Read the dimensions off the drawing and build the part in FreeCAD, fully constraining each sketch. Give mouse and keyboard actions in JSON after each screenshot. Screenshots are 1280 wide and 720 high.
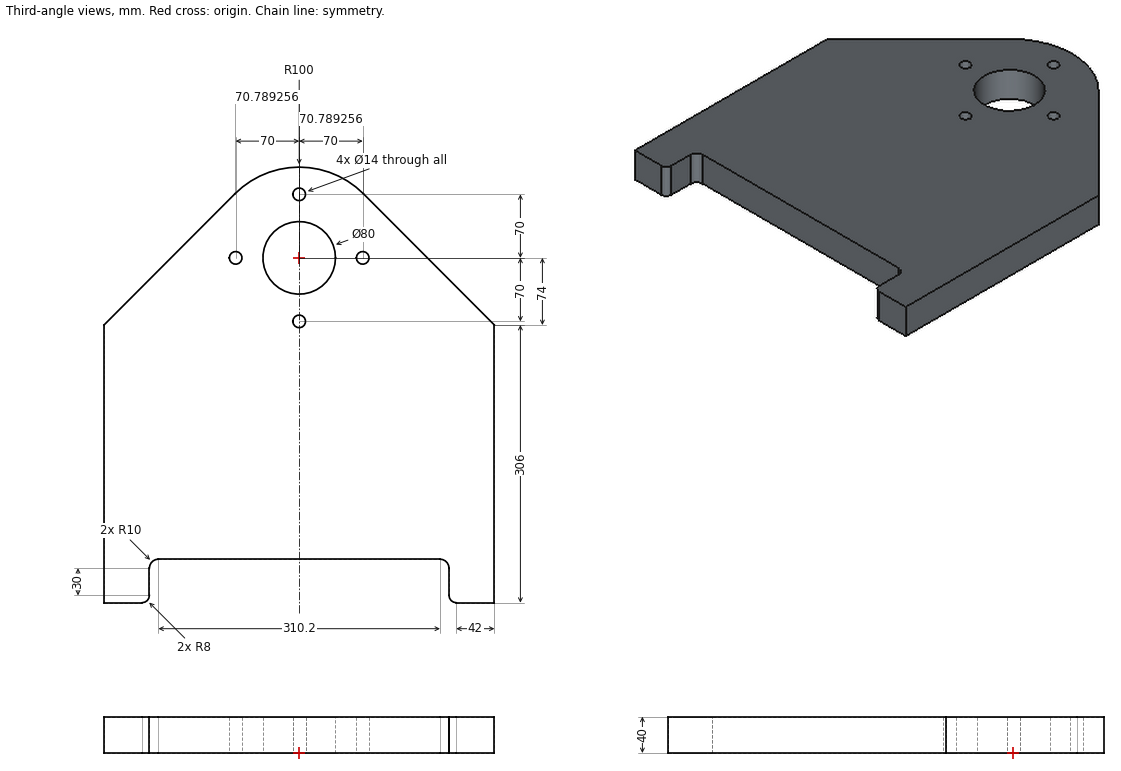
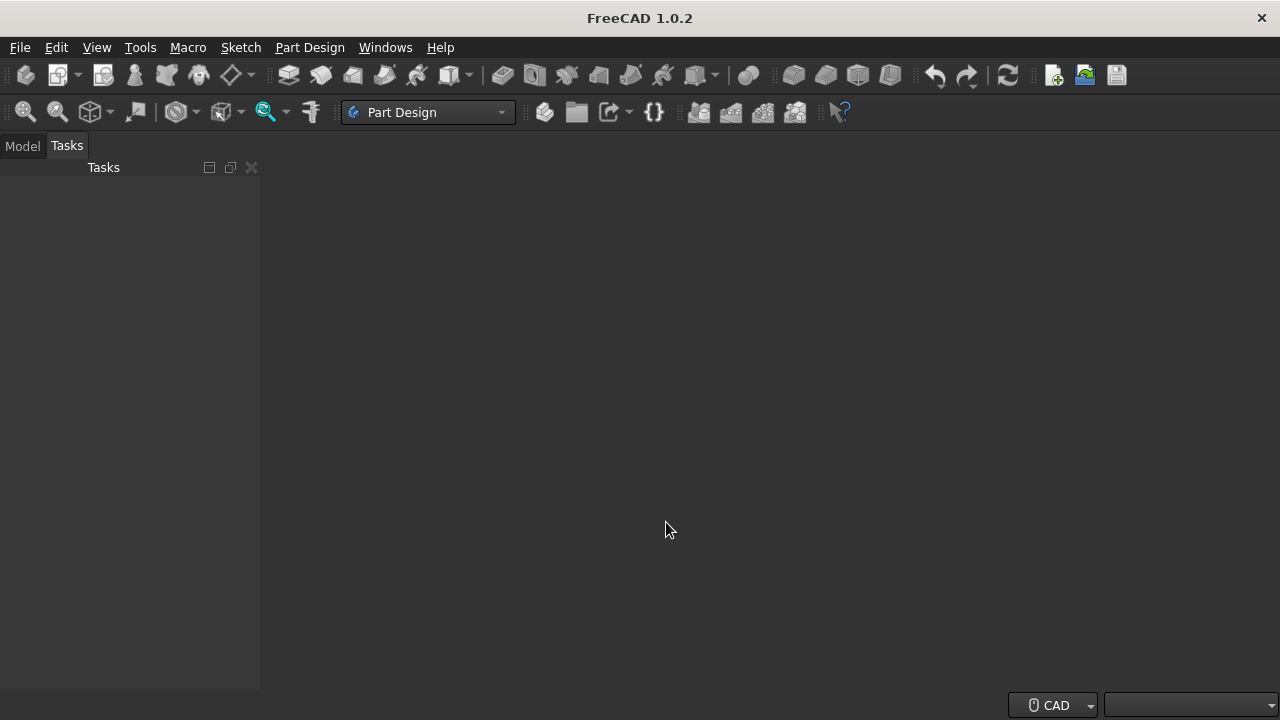
{"action": "key", "text": "ctrl+n"}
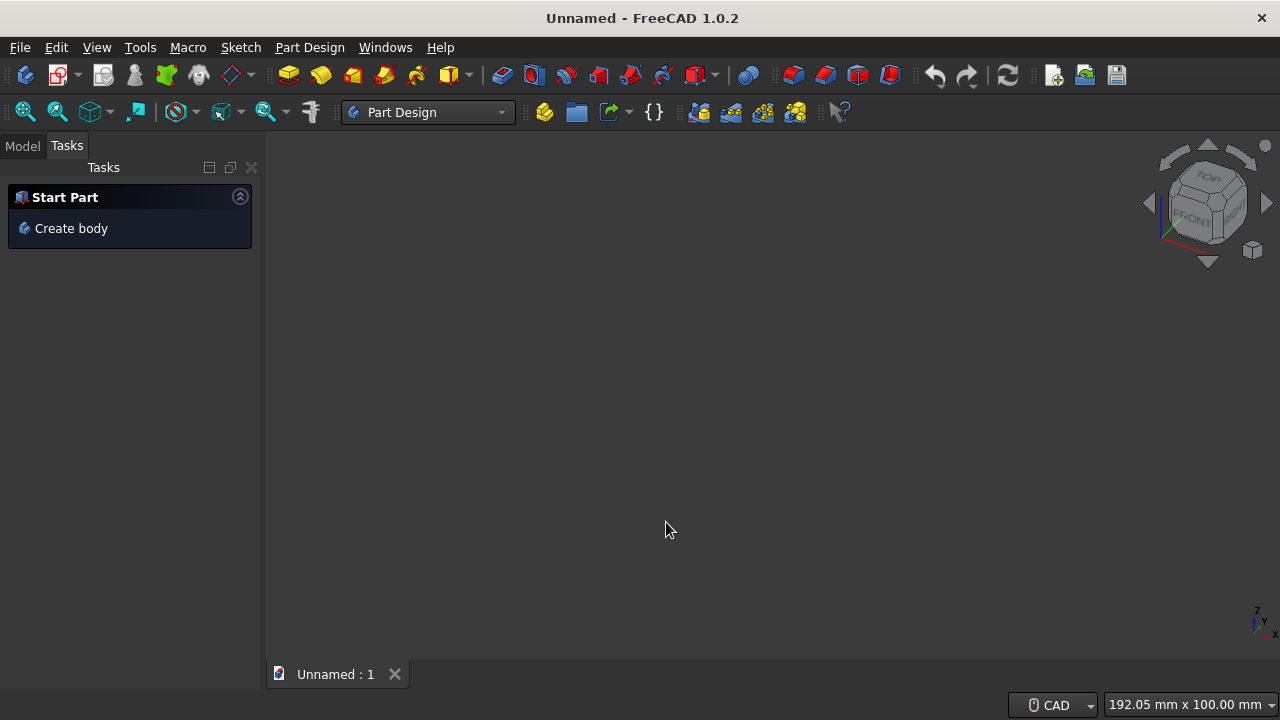
{"action": "left_click", "coordinate": [58, 76]}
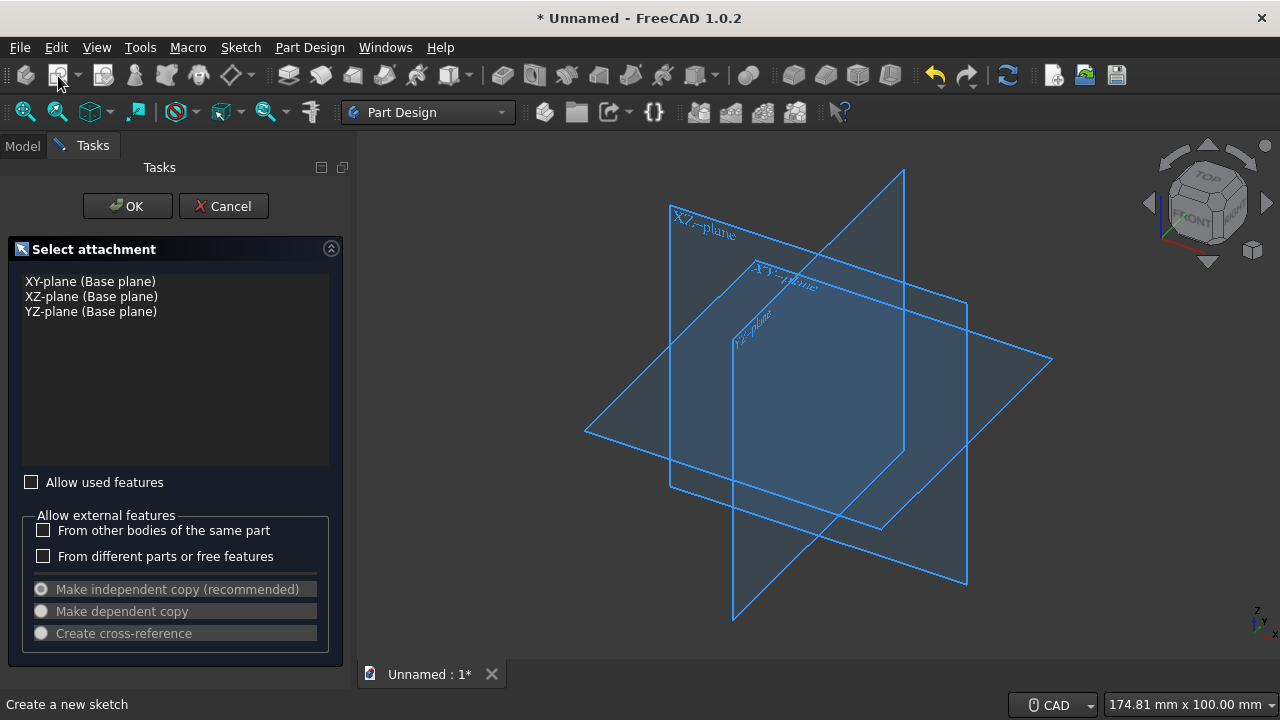
{"action": "left_click", "coordinate": [82, 282]}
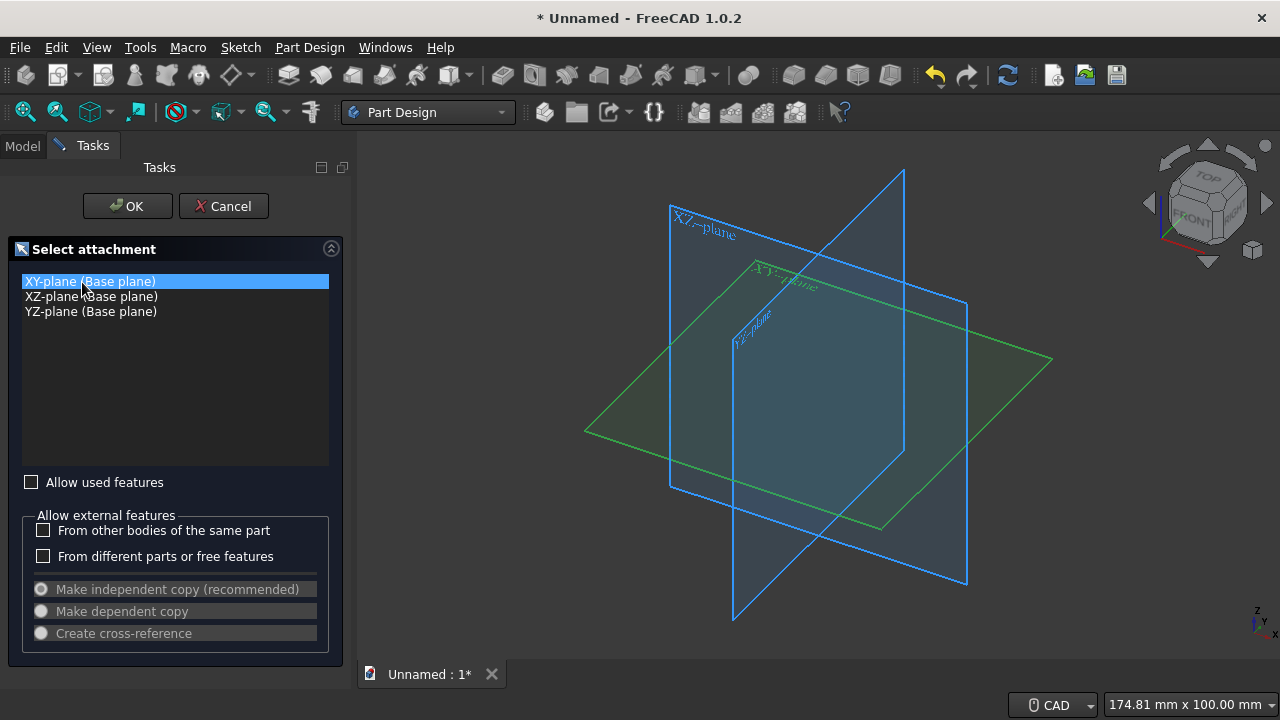
{"action": "left_click", "coordinate": [128, 206]}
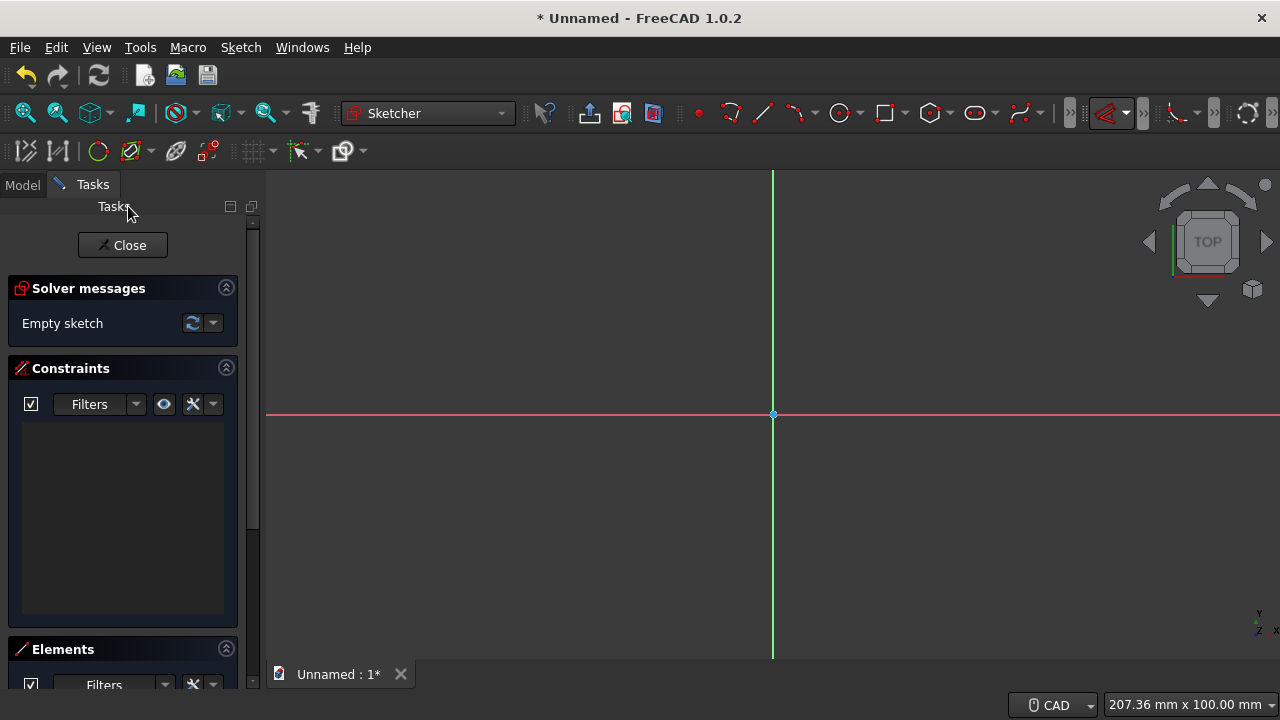
{"action": "scroll", "coordinate": [694, 307], "scroll_direction": "down", "scroll_amount": 10}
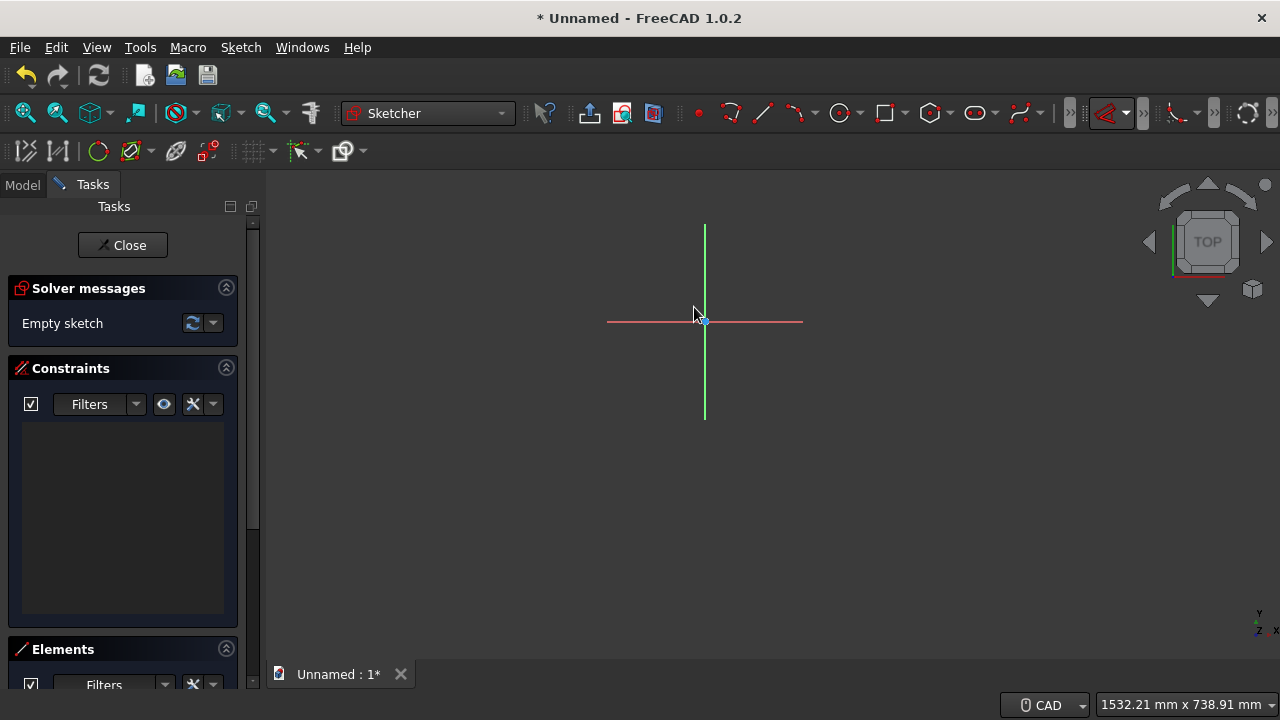
{"action": "key", "text": "g l"}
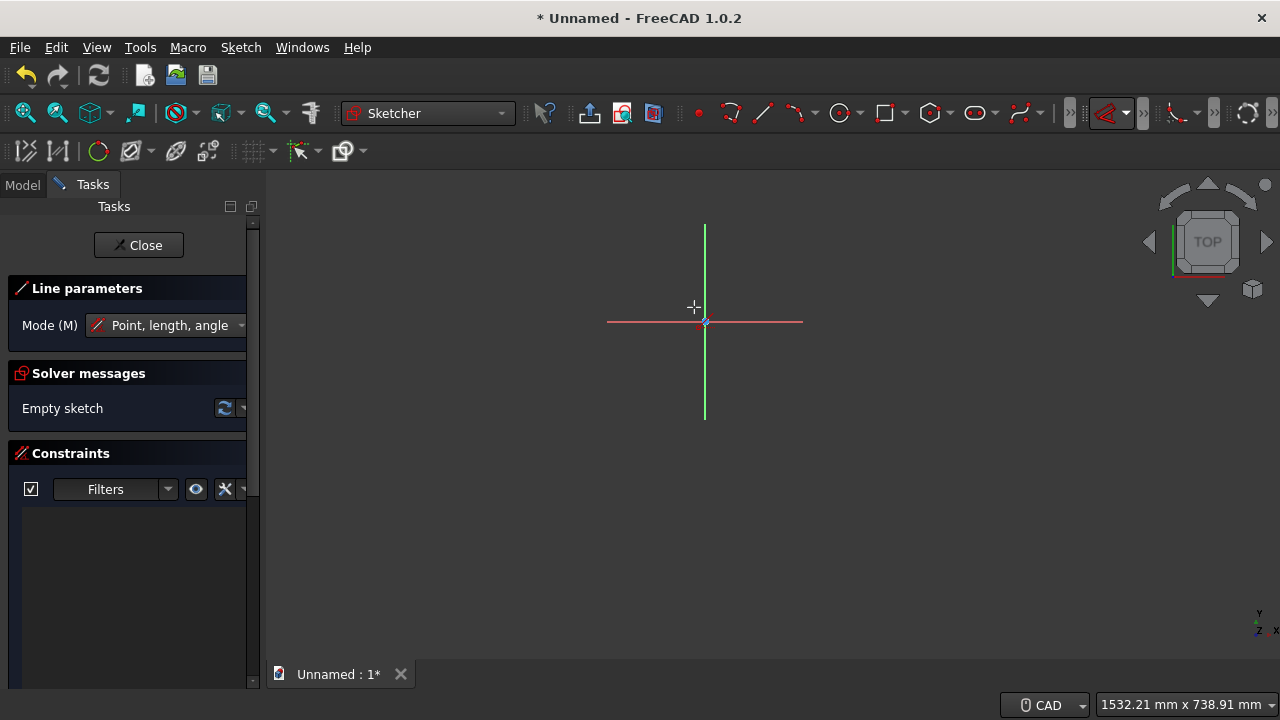
{"action": "left_click", "coordinate": [596, 568]}
{"action": "left_click", "coordinate": [596, 548]}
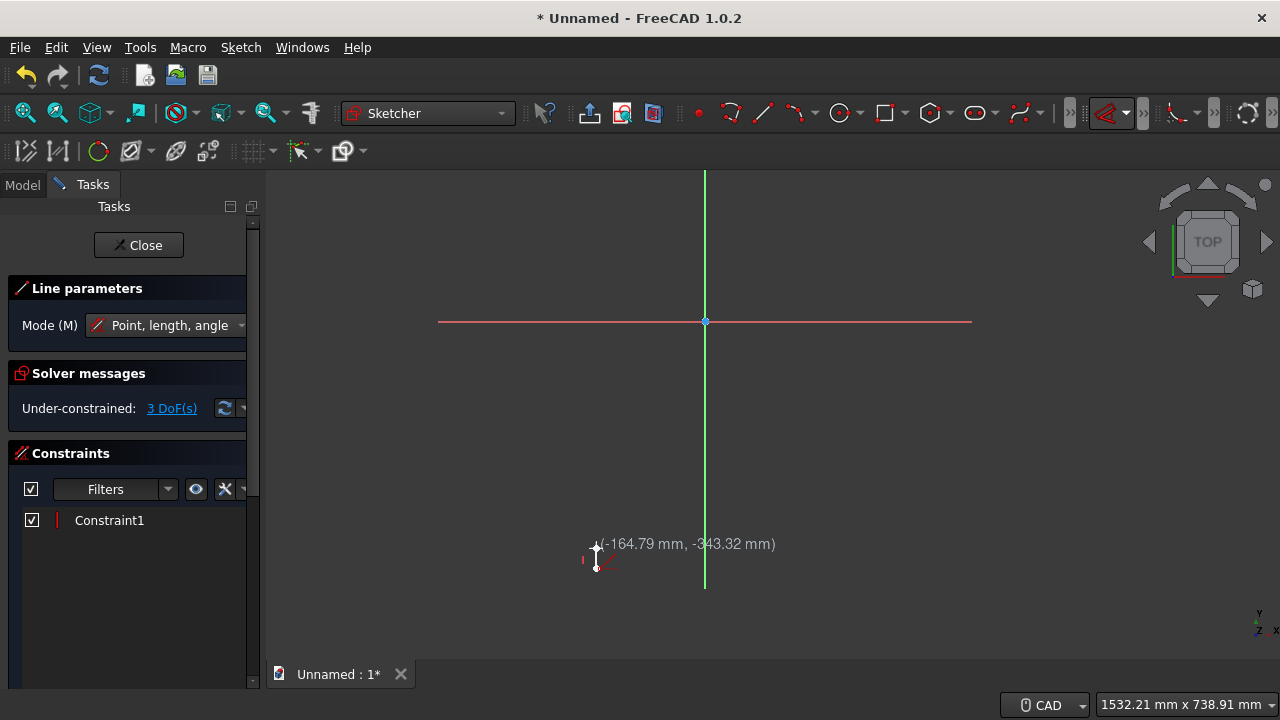
{"action": "scroll", "coordinate": [602, 542], "scroll_direction": "up", "scroll_amount": 3}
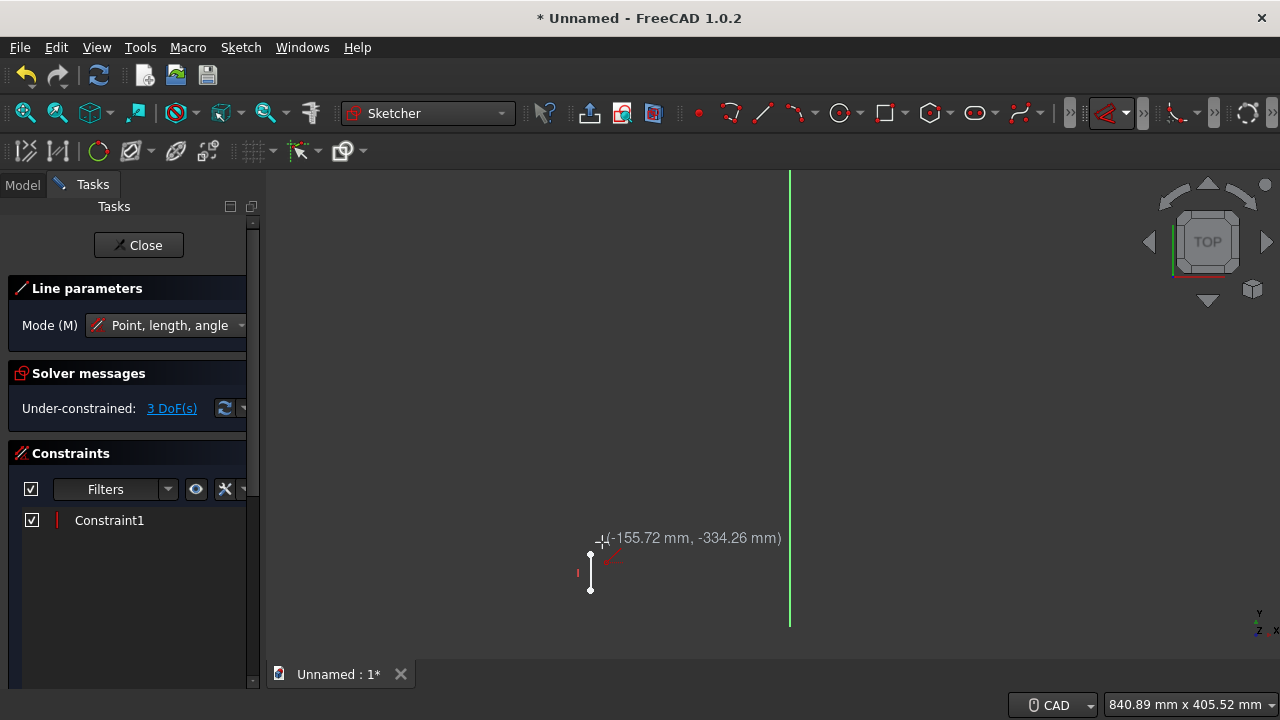
{"action": "left_click", "coordinate": [602, 540]}
{"action": "left_click", "coordinate": [977, 540]}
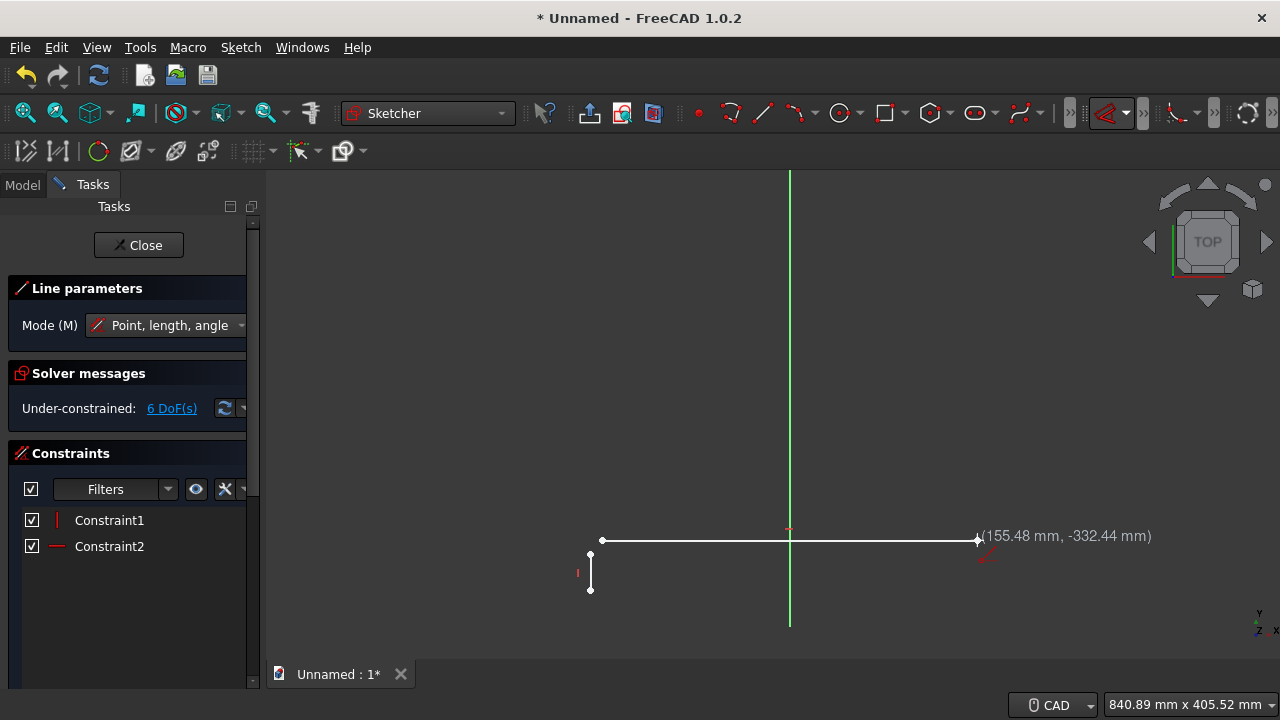
{"action": "left_click", "coordinate": [989, 553]}
{"action": "left_click", "coordinate": [989, 589]}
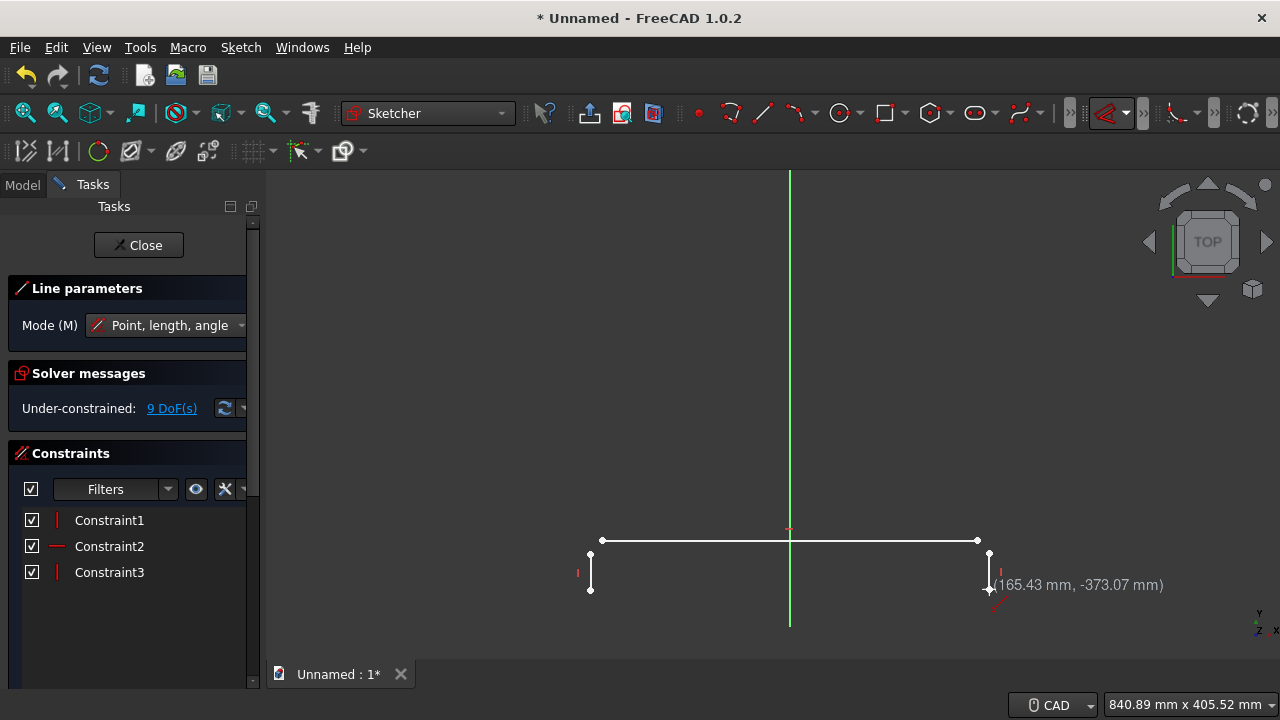
{"action": "key", "text": "g m"}